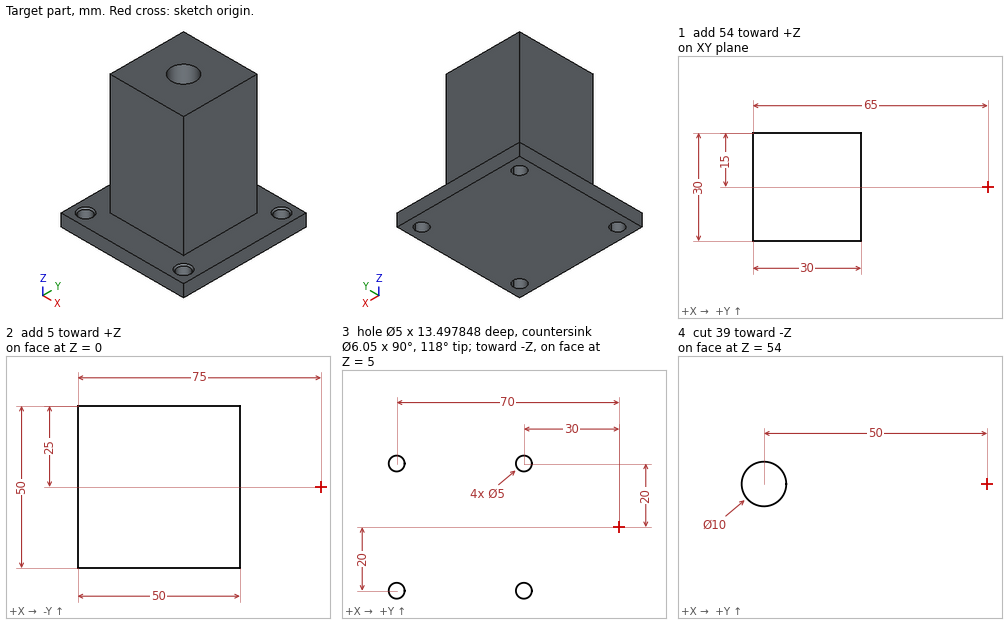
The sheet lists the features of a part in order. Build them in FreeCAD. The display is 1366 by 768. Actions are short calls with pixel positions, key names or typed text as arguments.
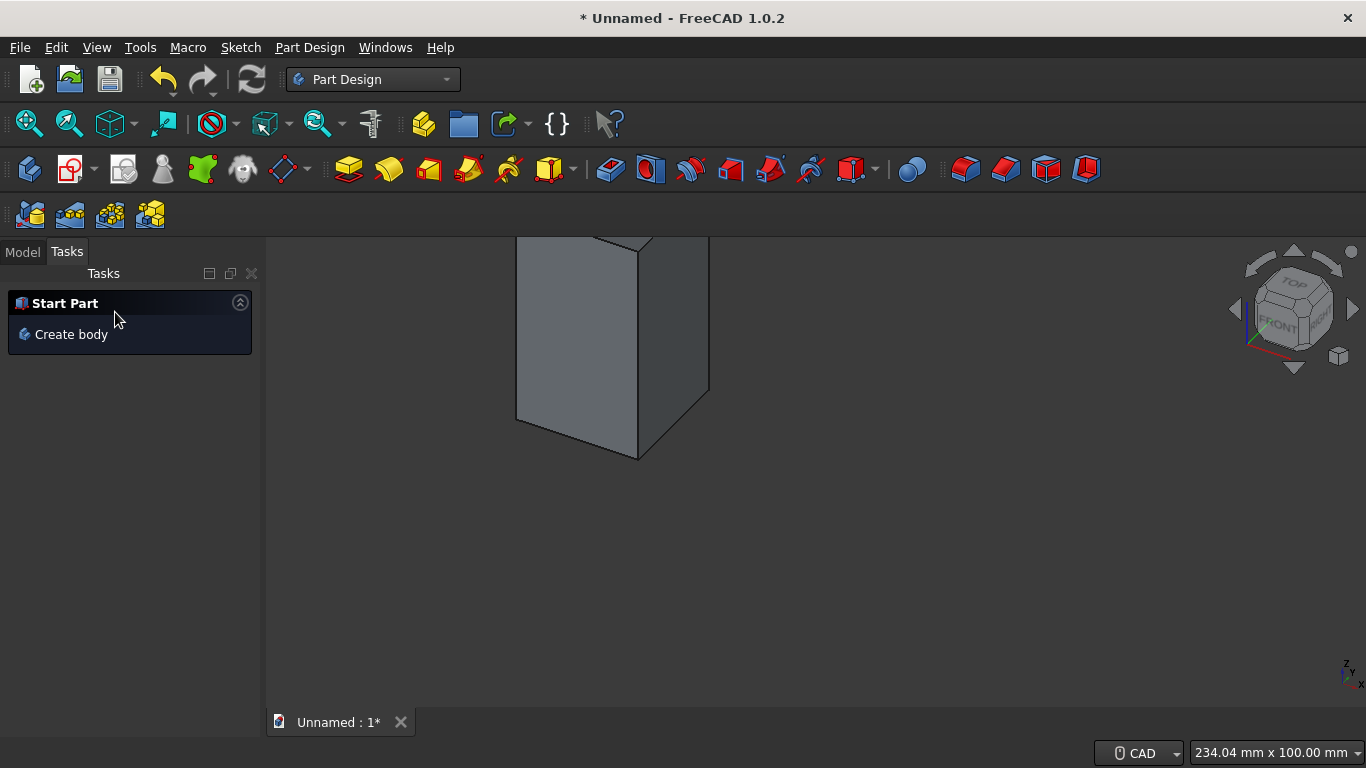
key(v)
key(f)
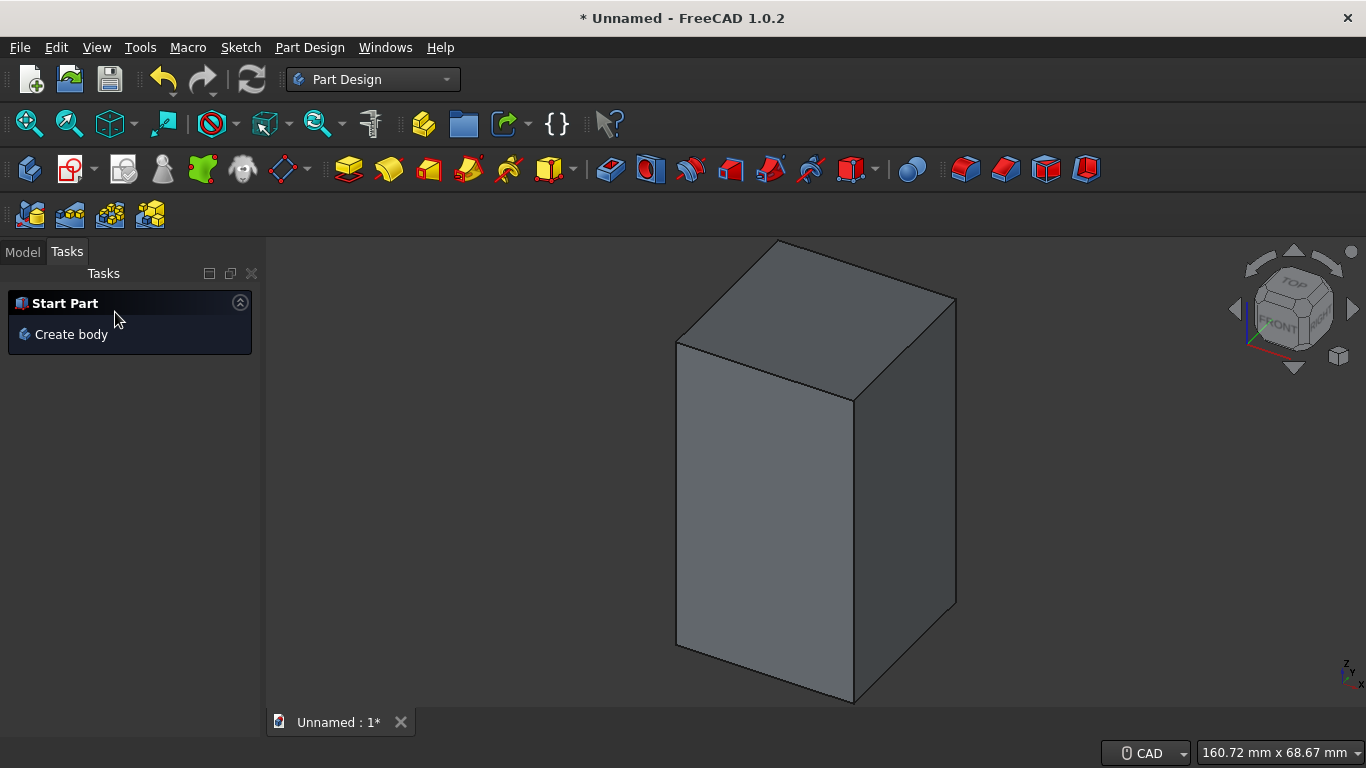
key(5)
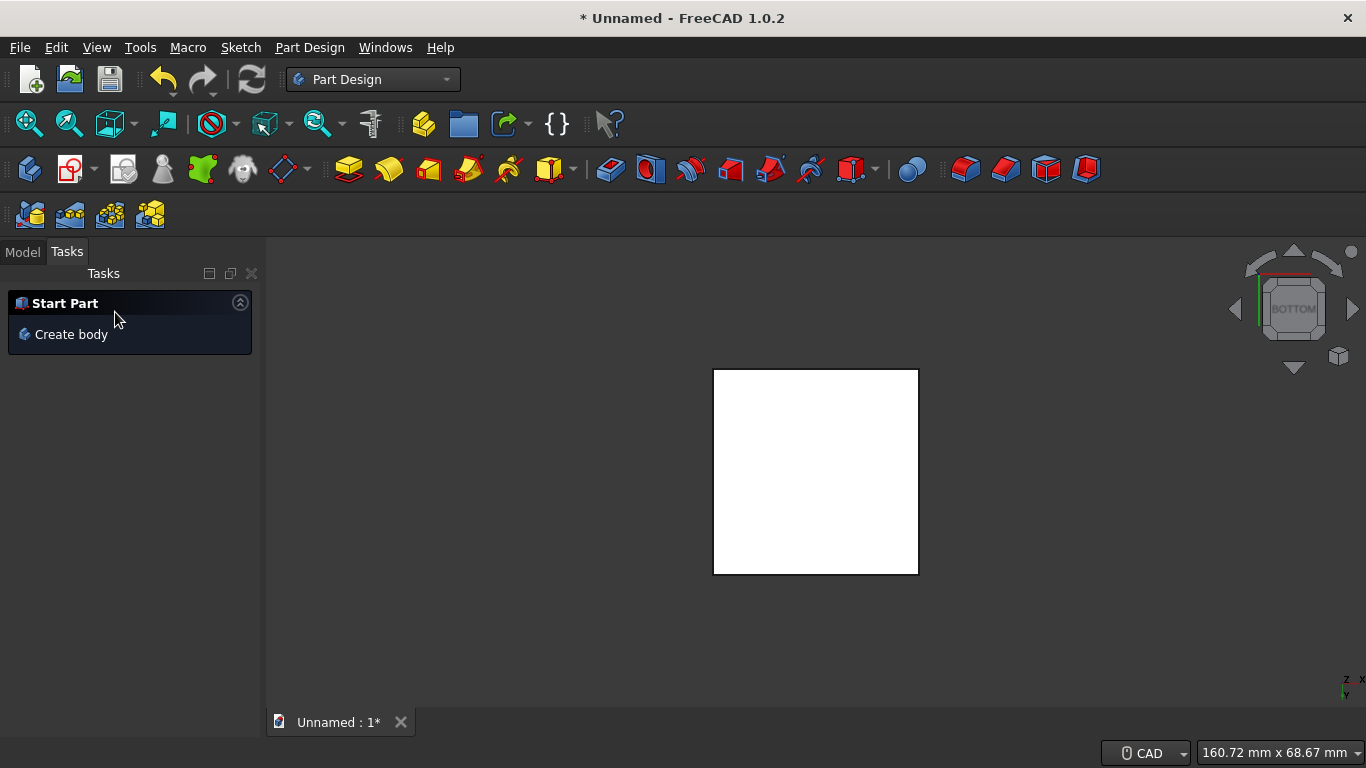
key(v)
key(f)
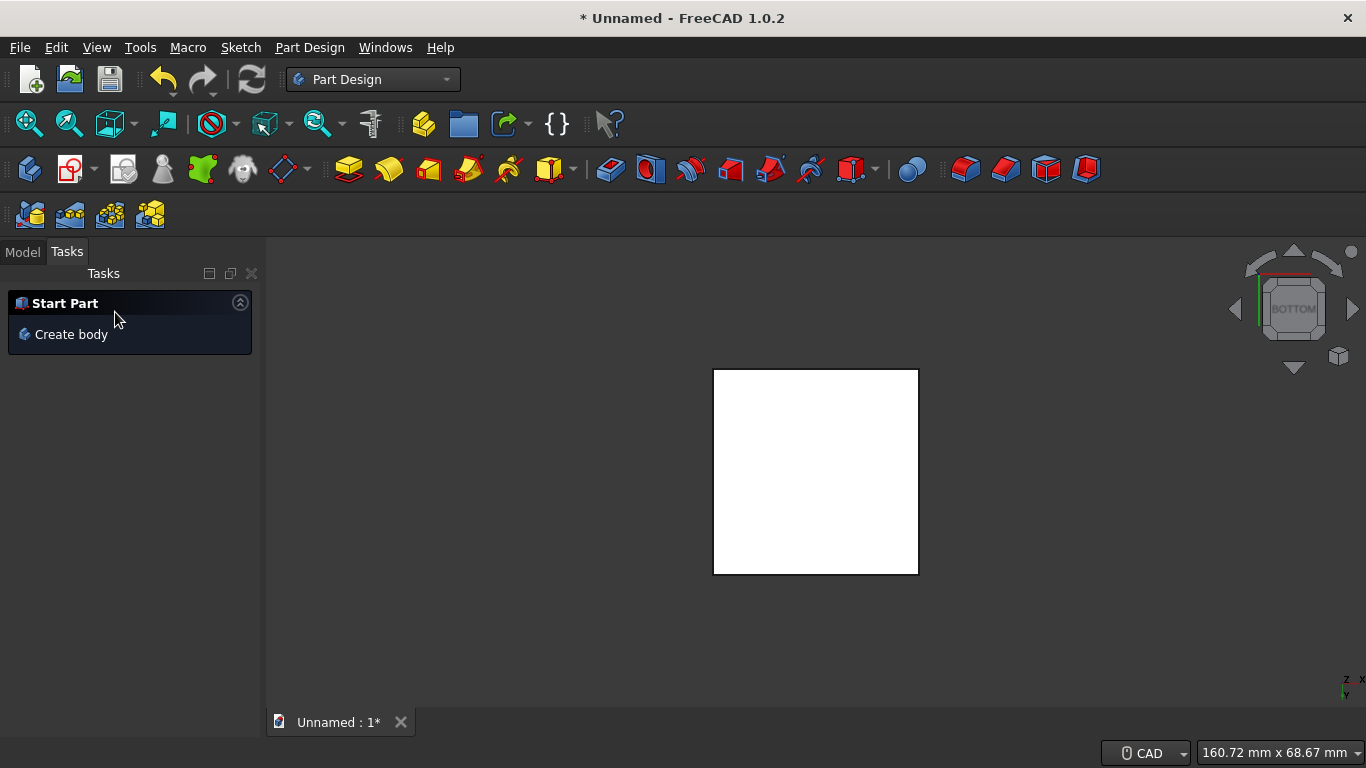
click(816, 471)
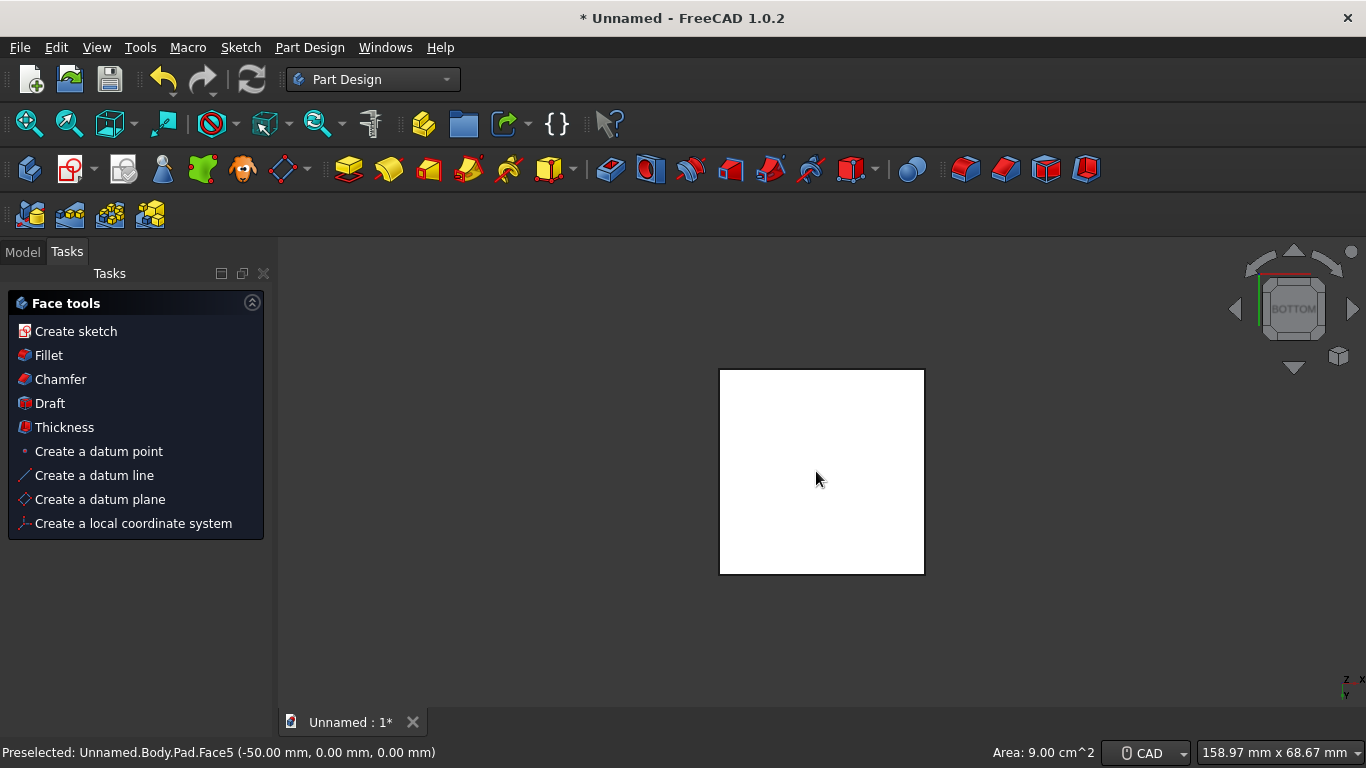
click(70, 170)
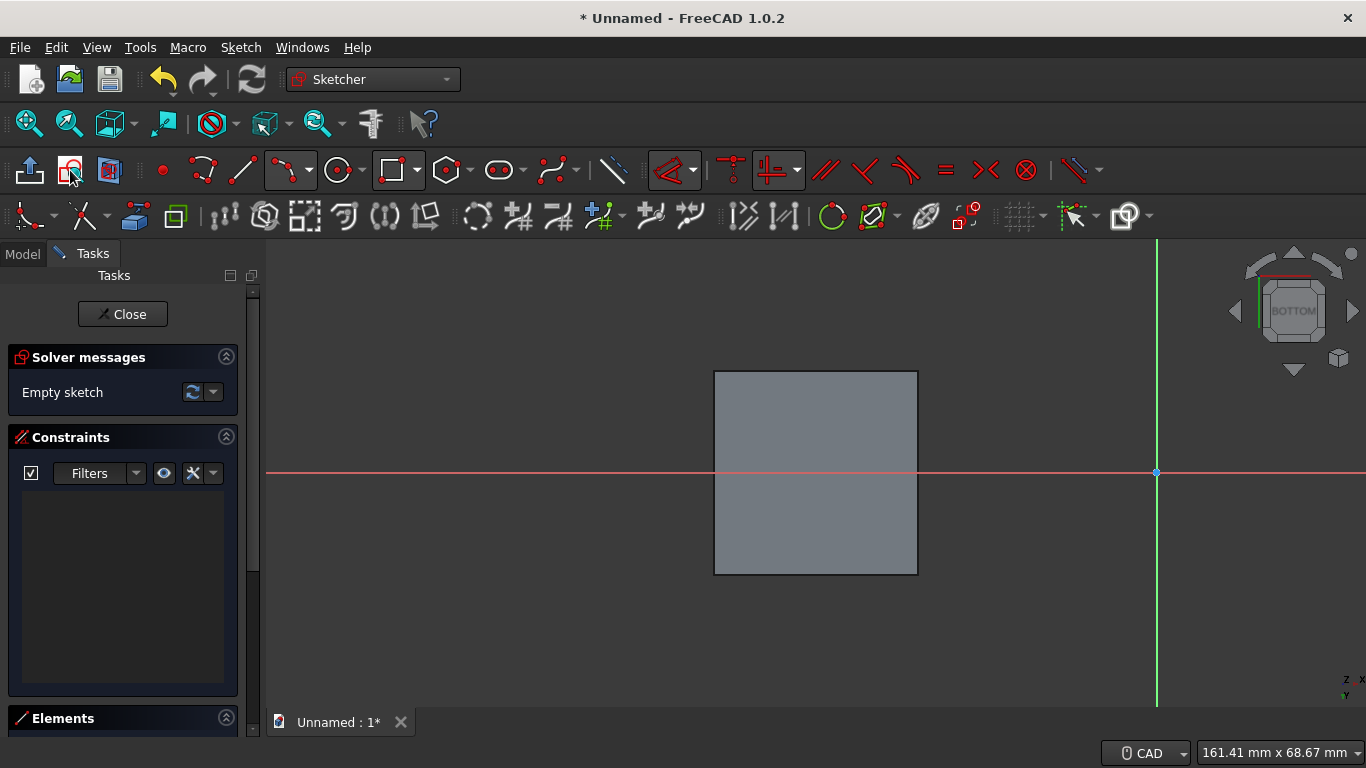
click(392, 170)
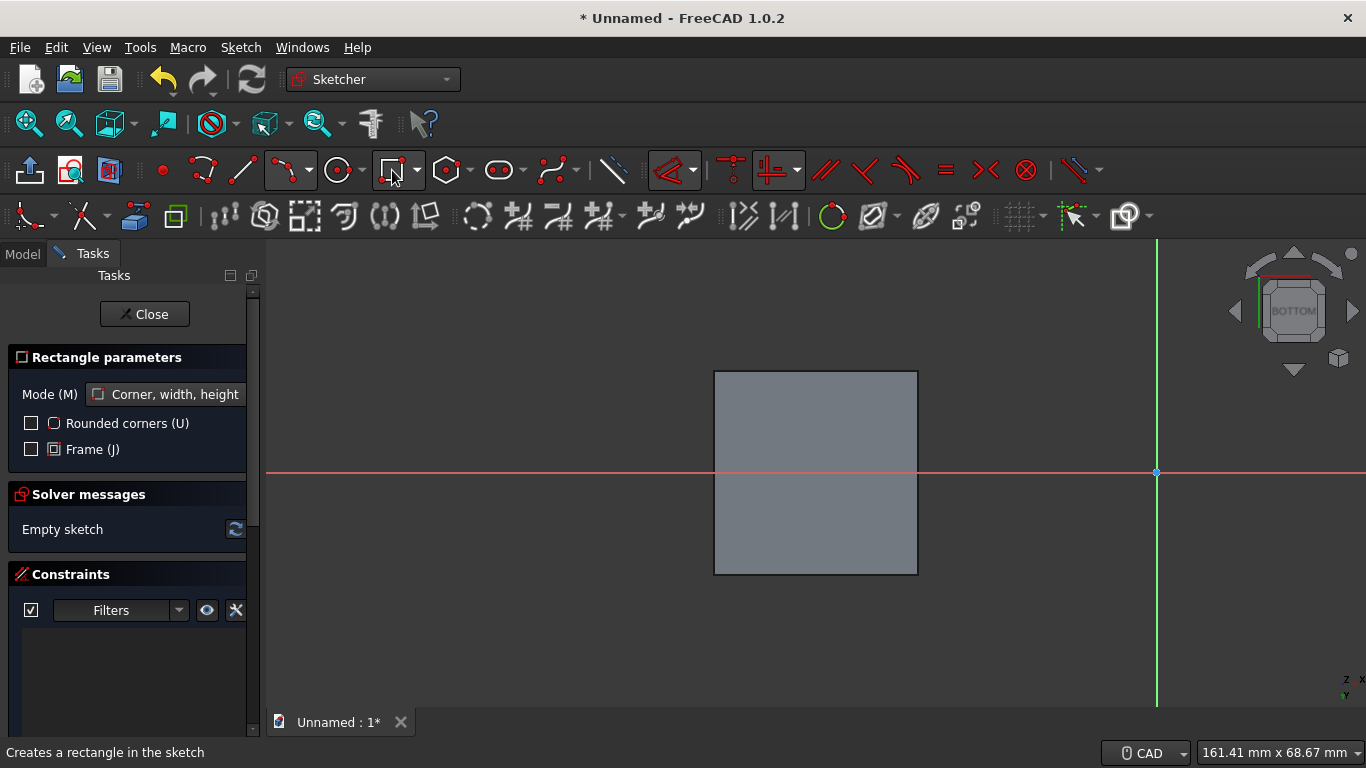
click(646, 303)
click(986, 643)
key(Escape)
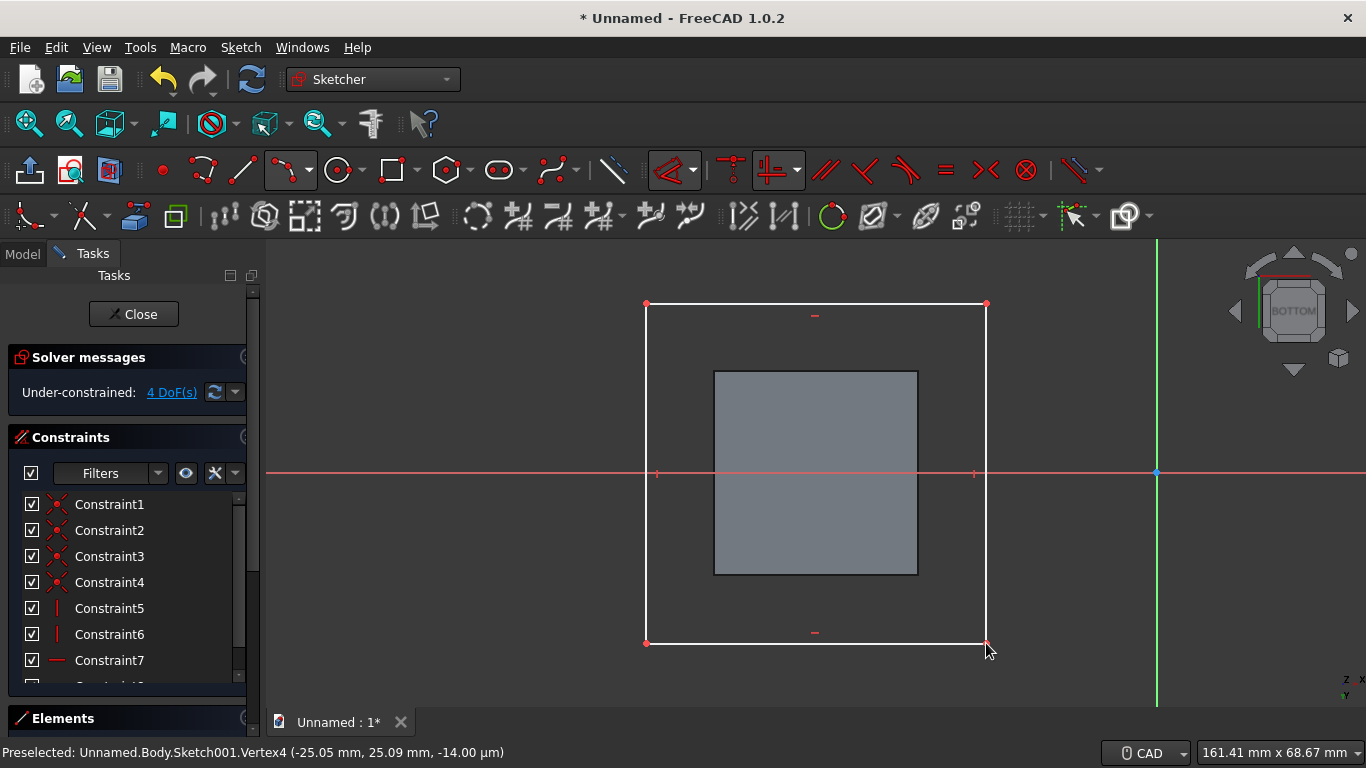
key(d)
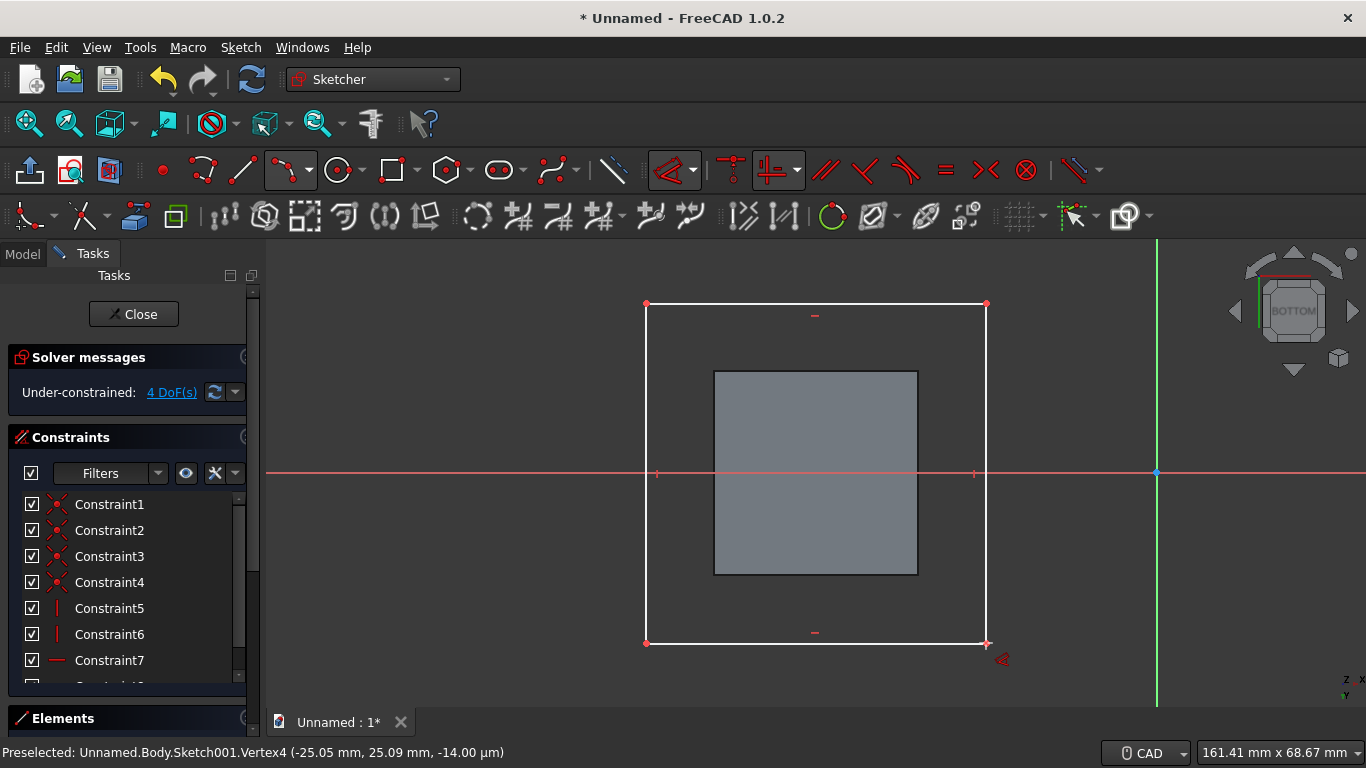
click(646, 406)
click(612, 396)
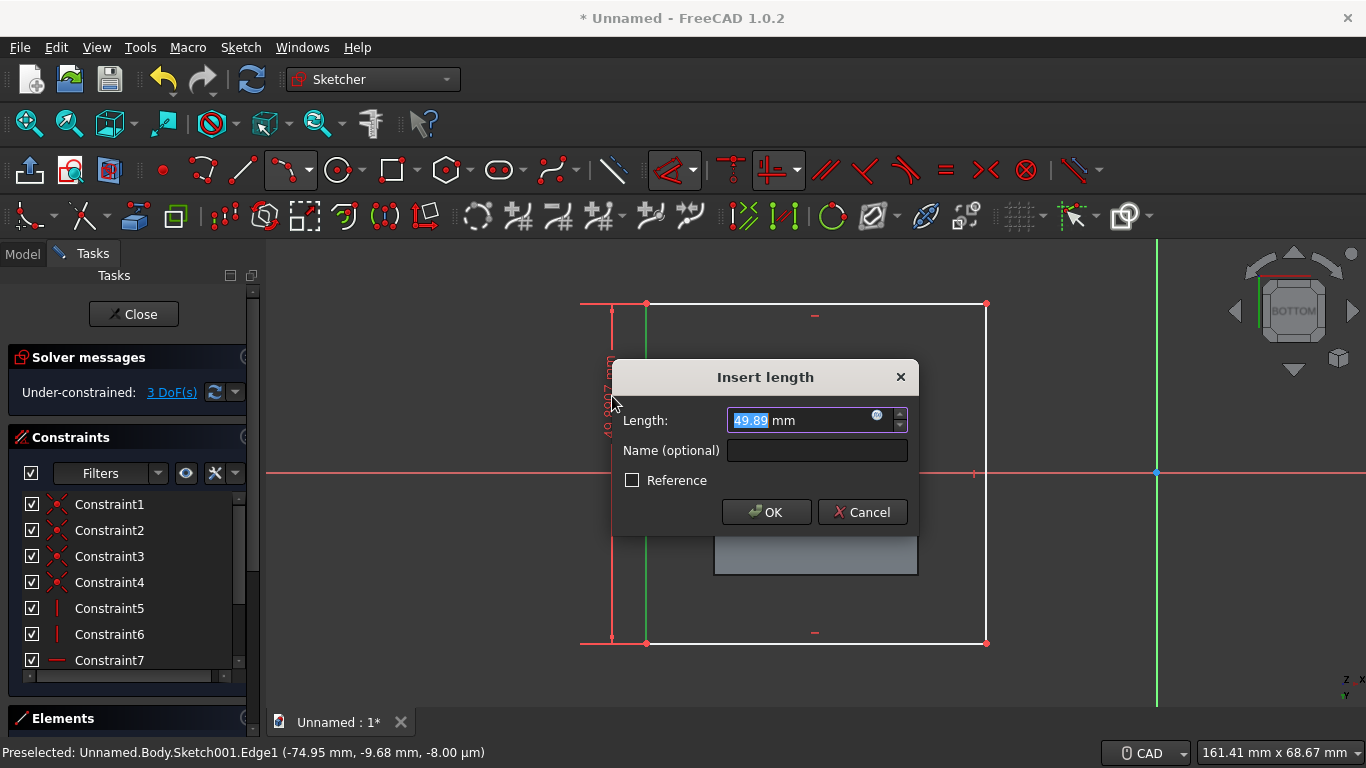
text(50)
key(Return)